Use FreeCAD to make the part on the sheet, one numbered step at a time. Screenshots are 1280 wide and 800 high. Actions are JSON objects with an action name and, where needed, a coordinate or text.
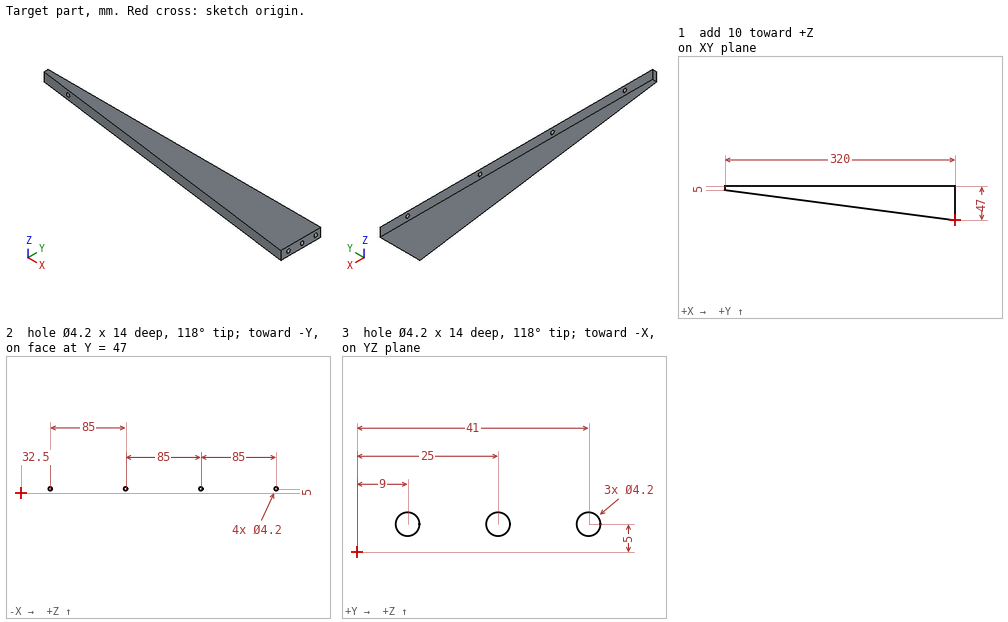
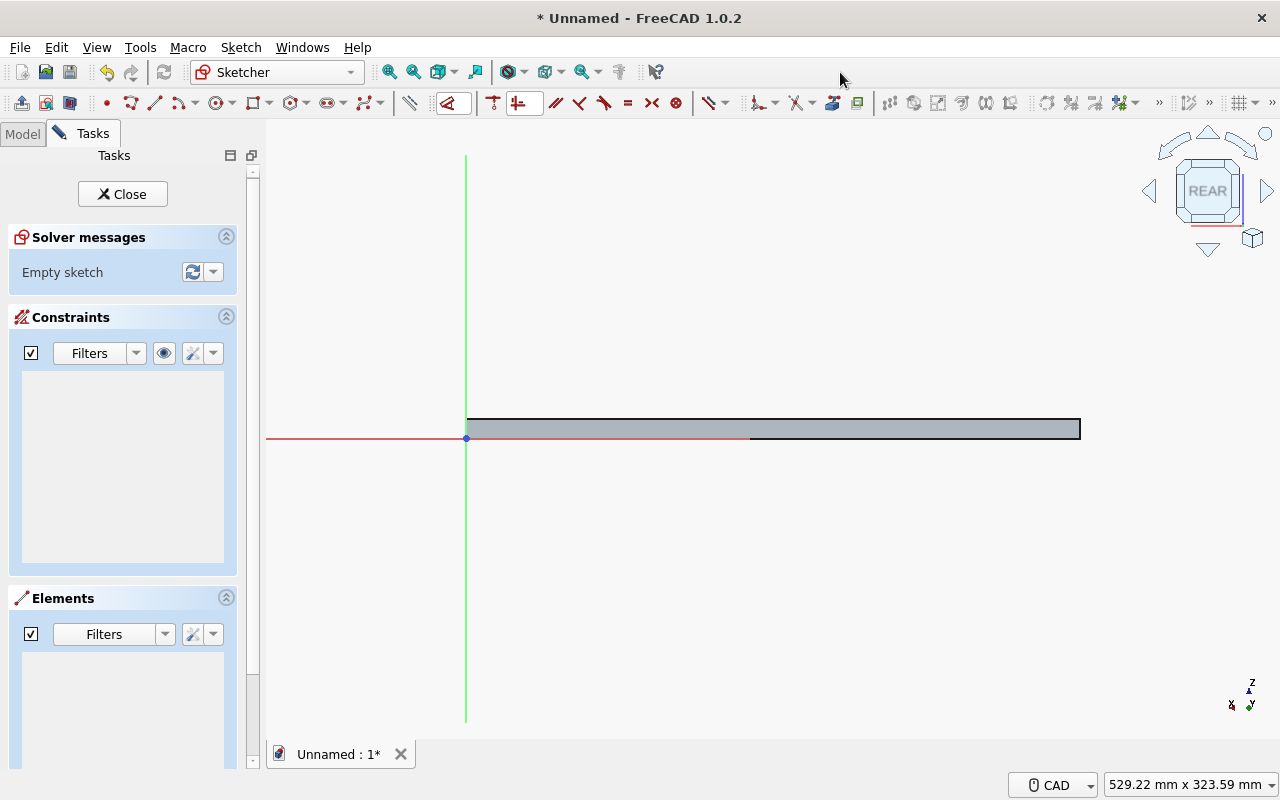
{"action": "left_click", "coordinate": [216, 104]}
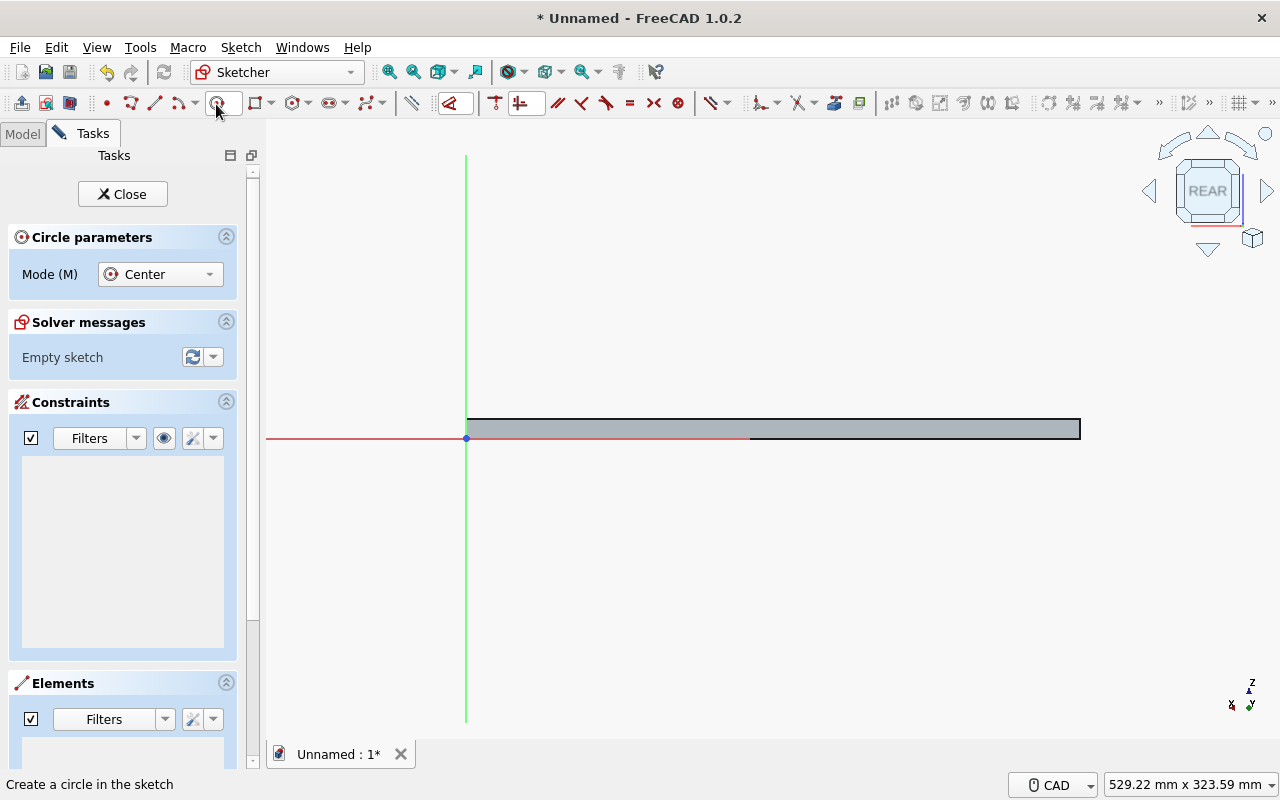
{"action": "scroll", "coordinate": [1017, 429], "scroll_direction": "up", "scroll_amount": 9}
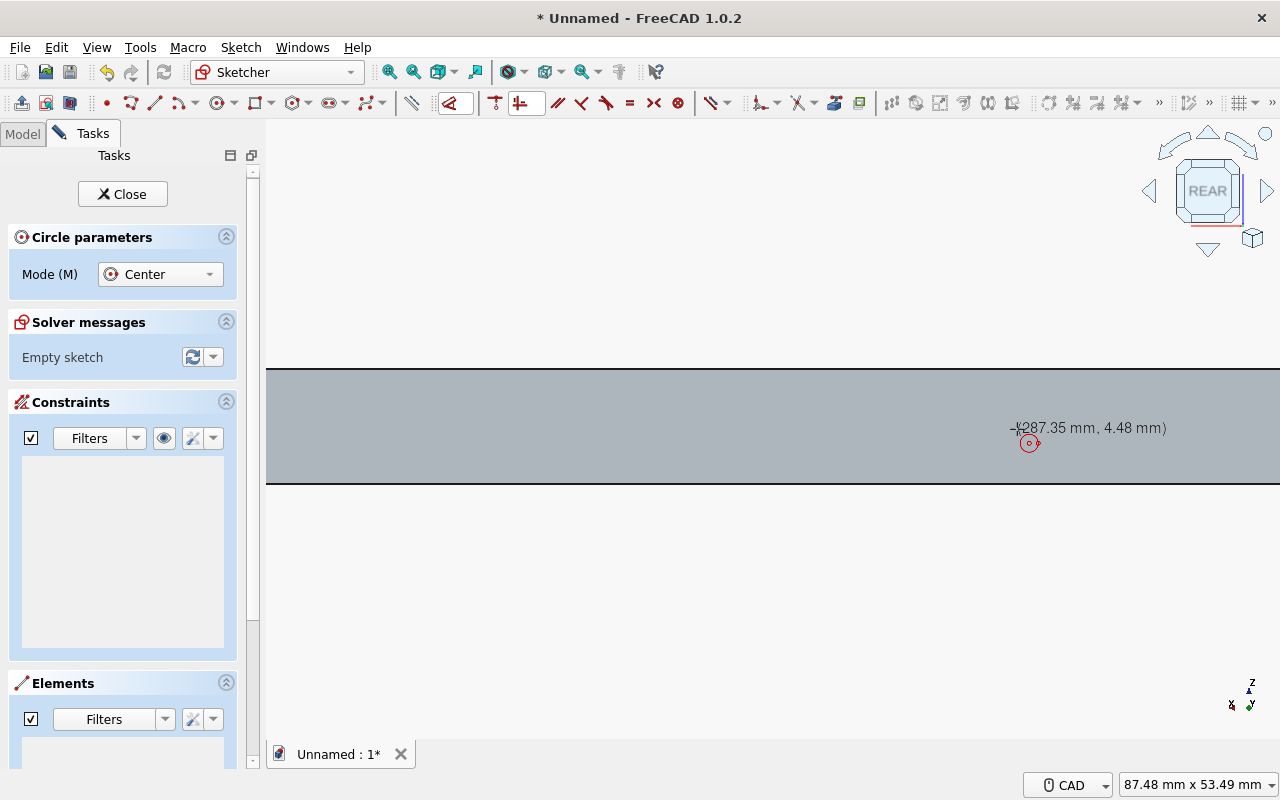
{"action": "scroll", "coordinate": [971, 426], "scroll_direction": "down", "scroll_amount": 9}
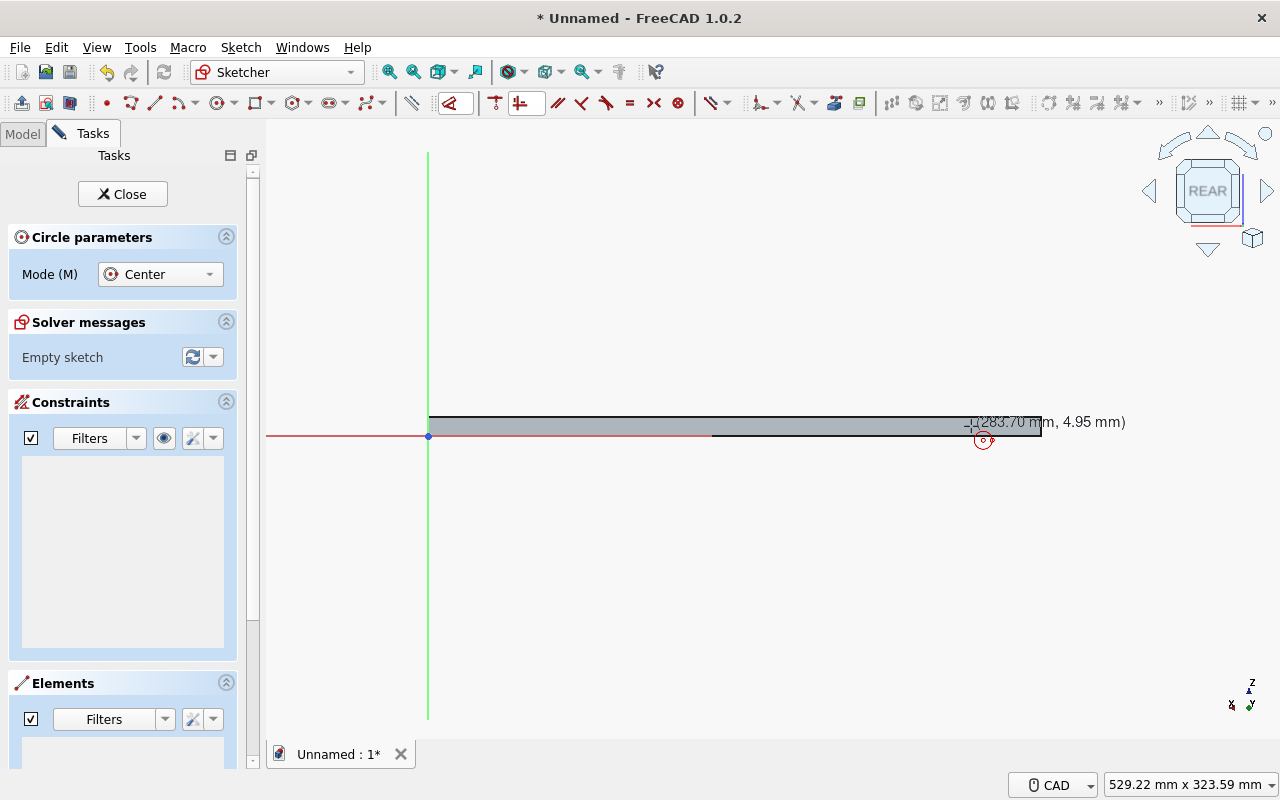
{"action": "scroll", "coordinate": [979, 426], "scroll_direction": "up", "scroll_amount": 3}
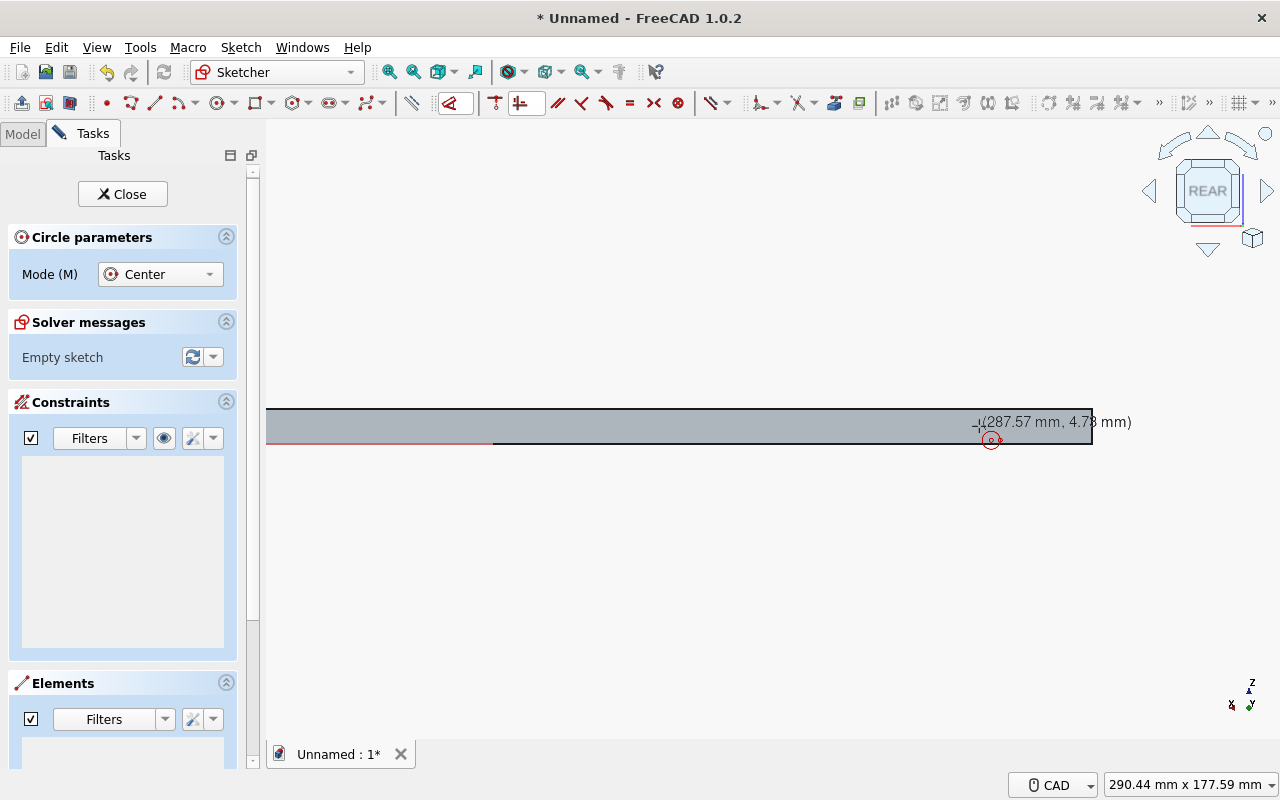
{"action": "left_click", "coordinate": [978, 426]}
{"action": "mouse_move", "coordinate": [983, 421]}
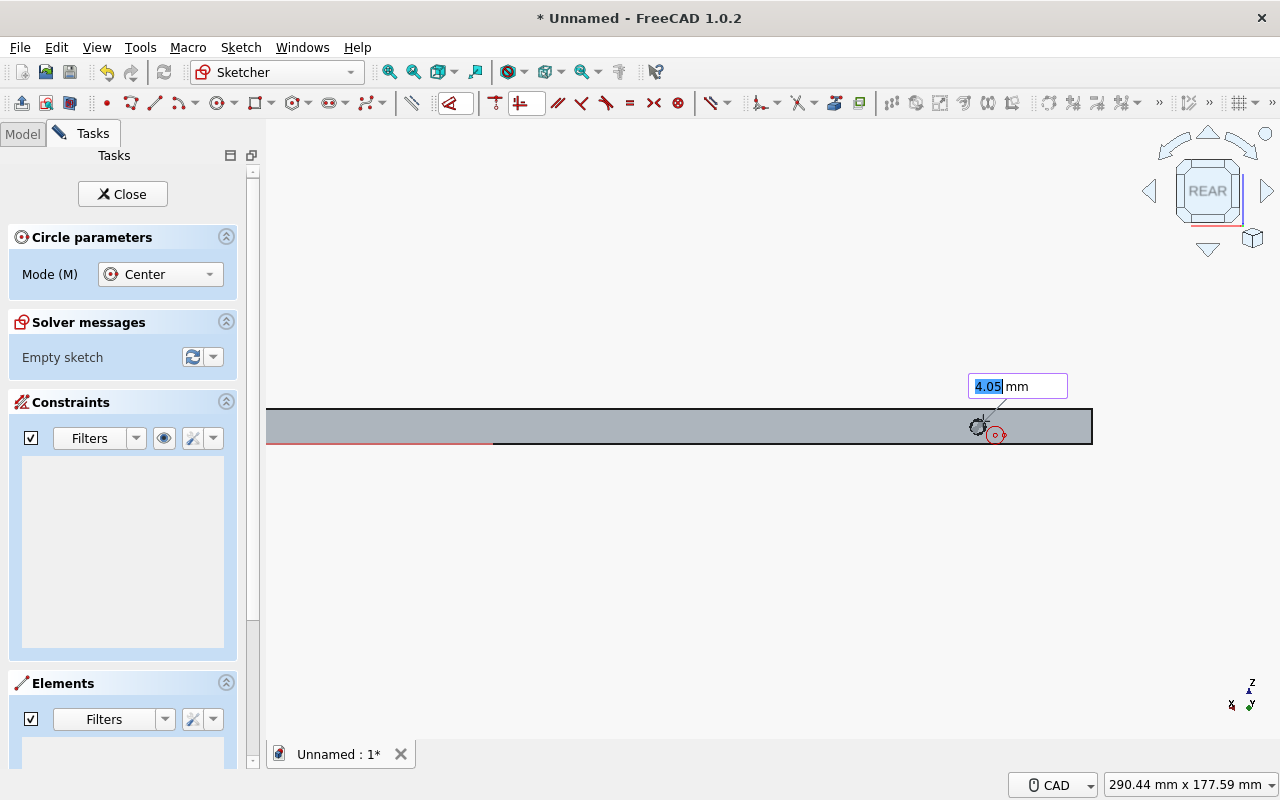
{"action": "type", "text": "4.2"}
{"action": "key", "text": "Return"}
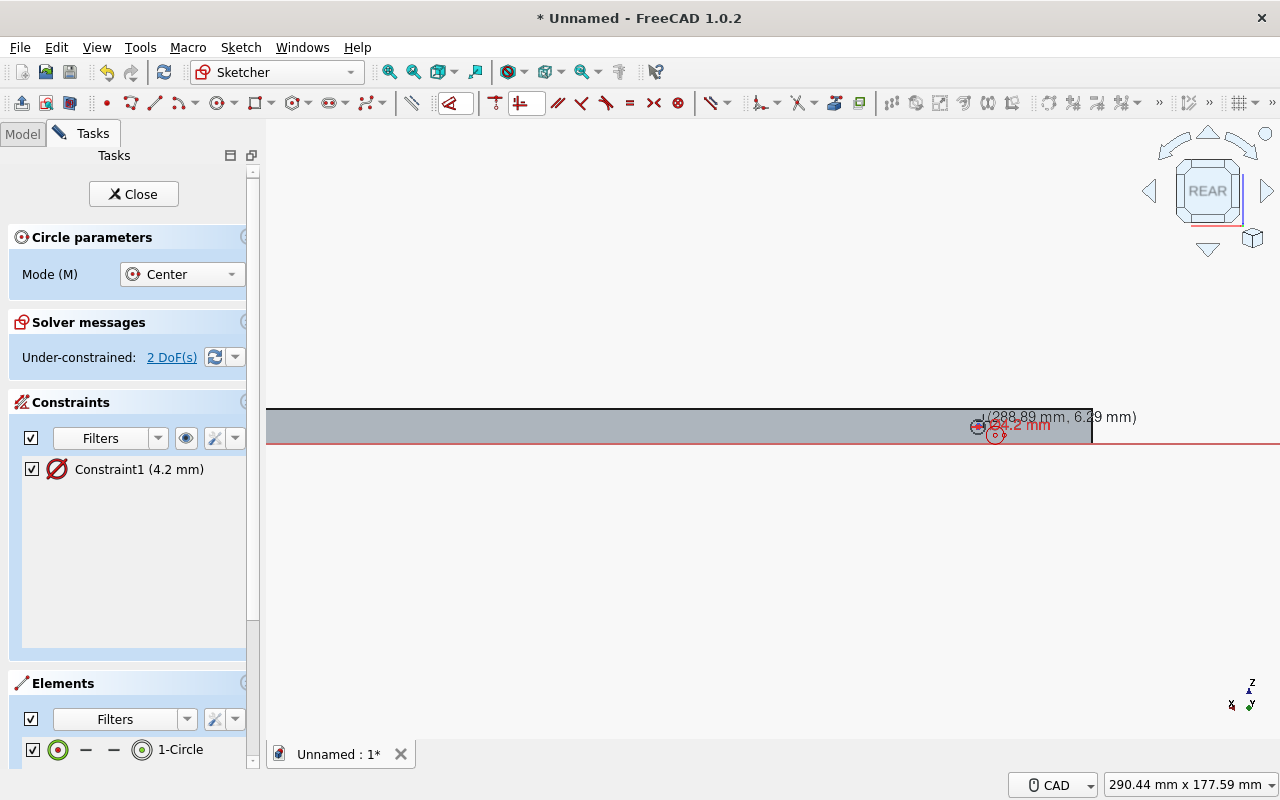
{"action": "scroll", "coordinate": [681, 426], "scroll_direction": "up", "scroll_amount": 6}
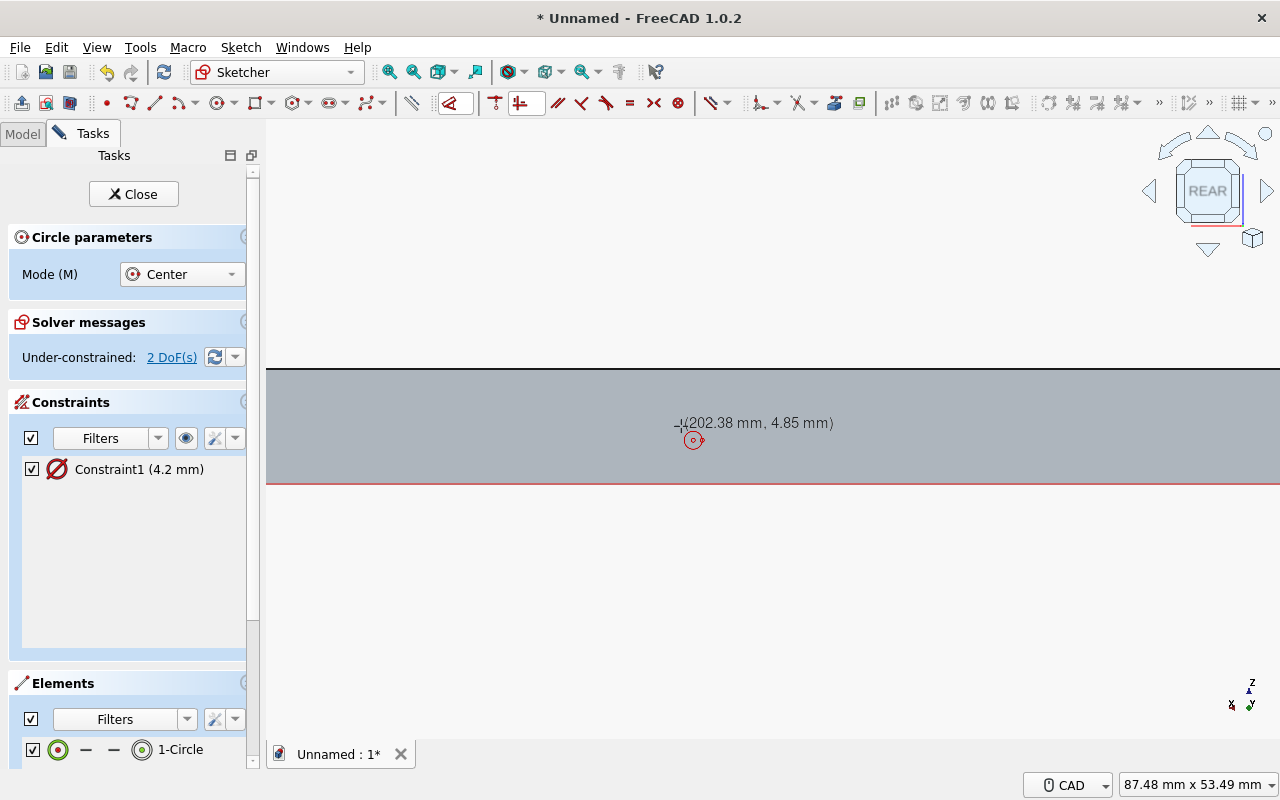
{"action": "scroll", "coordinate": [842, 426], "scroll_direction": "down", "scroll_amount": 9}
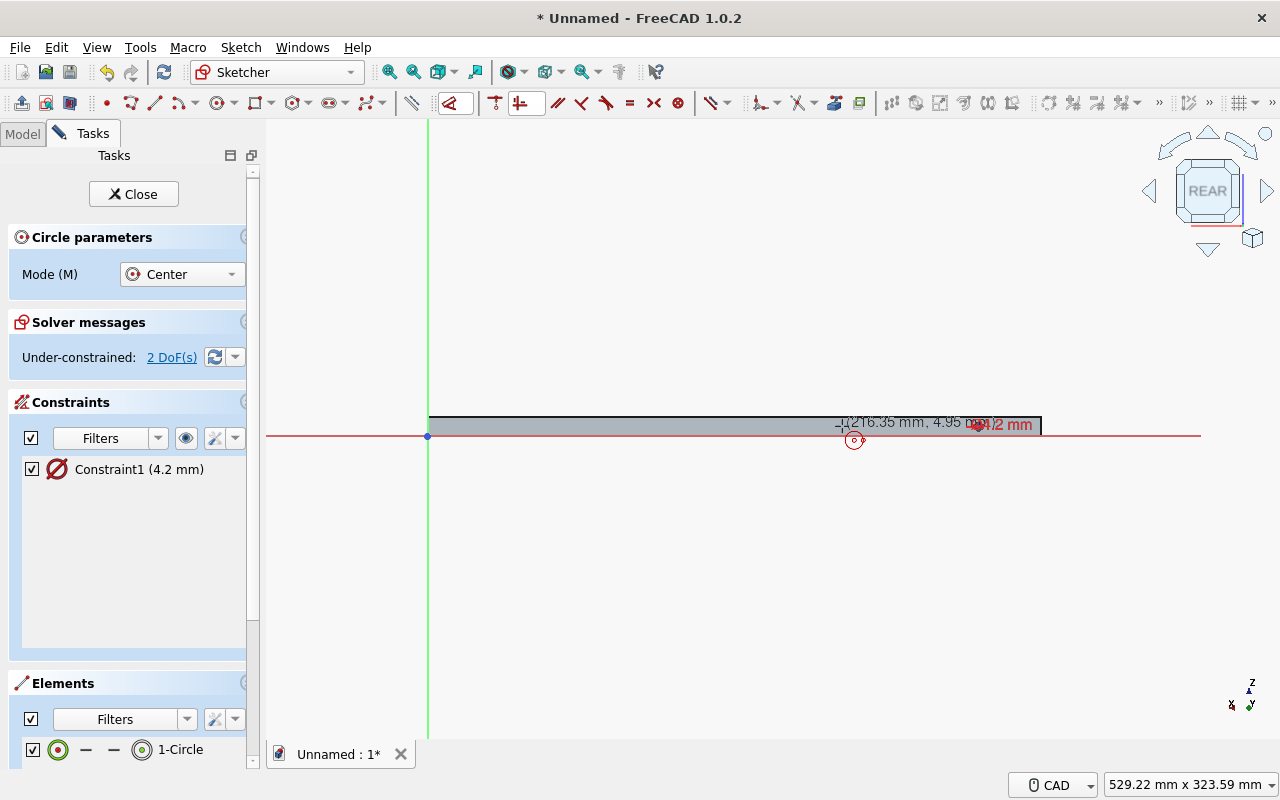
{"action": "scroll", "coordinate": [816, 426], "scroll_direction": "up", "scroll_amount": 3}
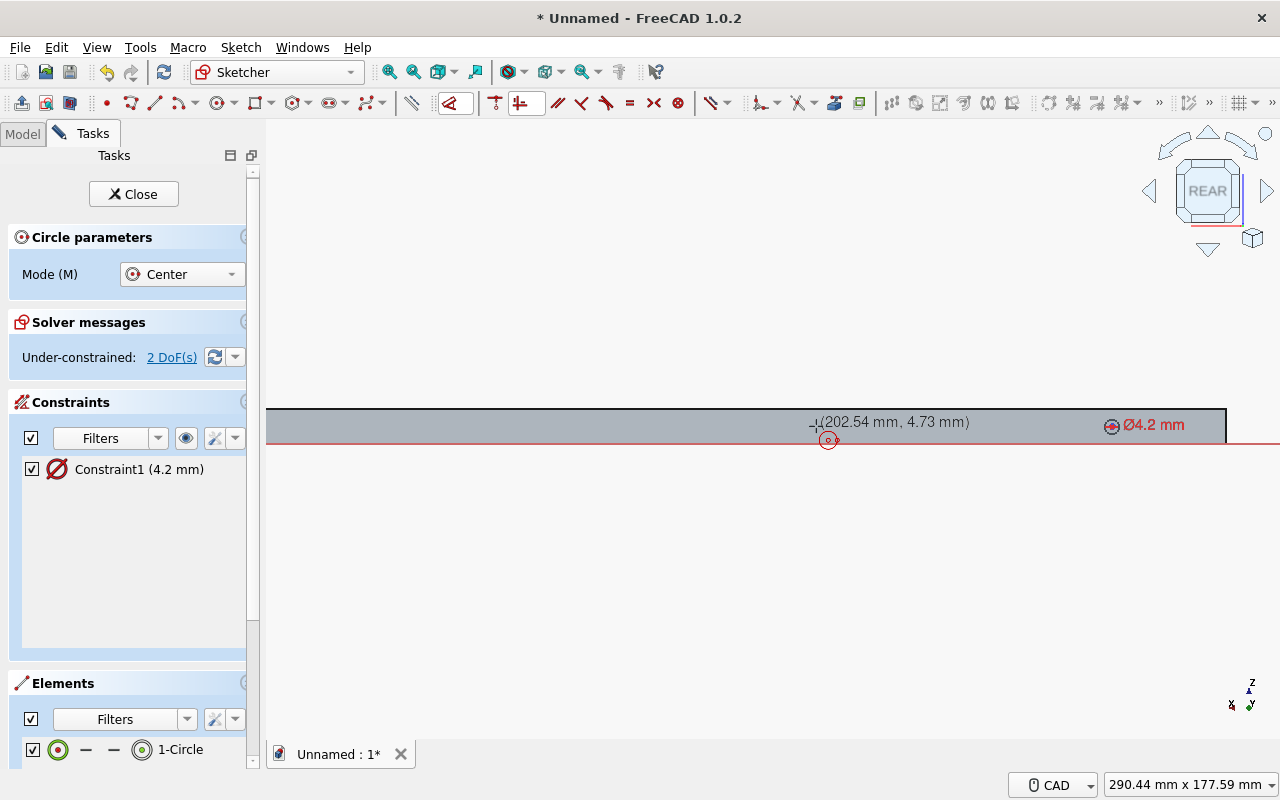
{"action": "left_click", "coordinate": [815, 426]}
{"action": "mouse_move", "coordinate": [821, 421]}